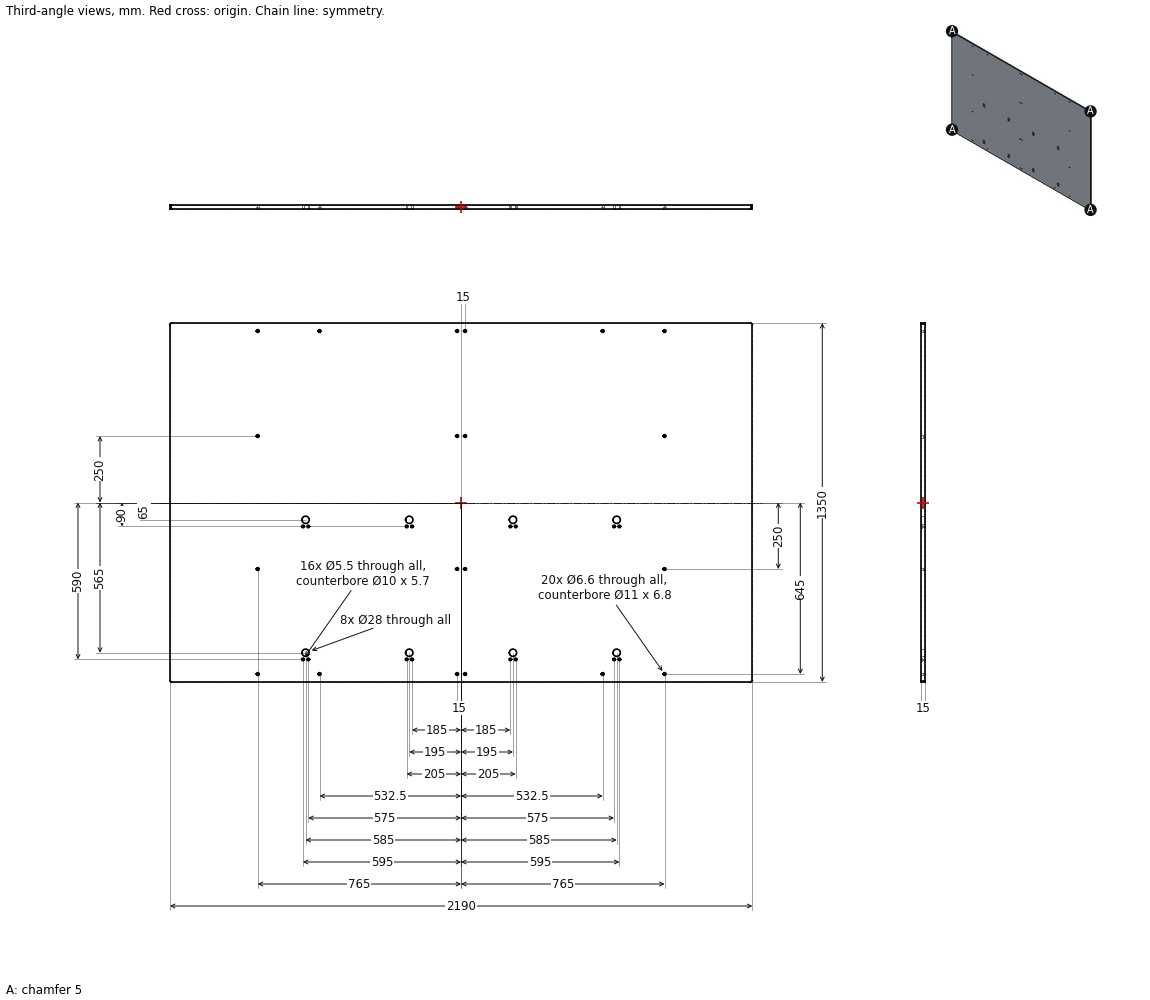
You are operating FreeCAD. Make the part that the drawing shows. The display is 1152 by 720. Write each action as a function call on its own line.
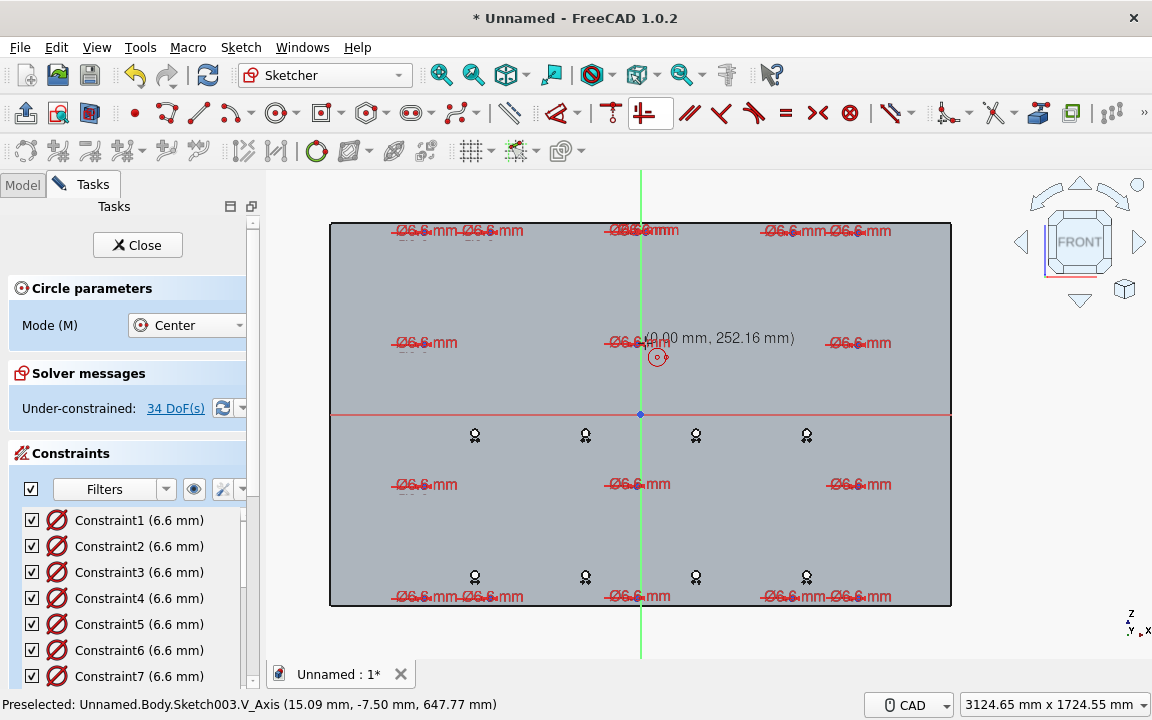
scroll(645, 344, up, 7)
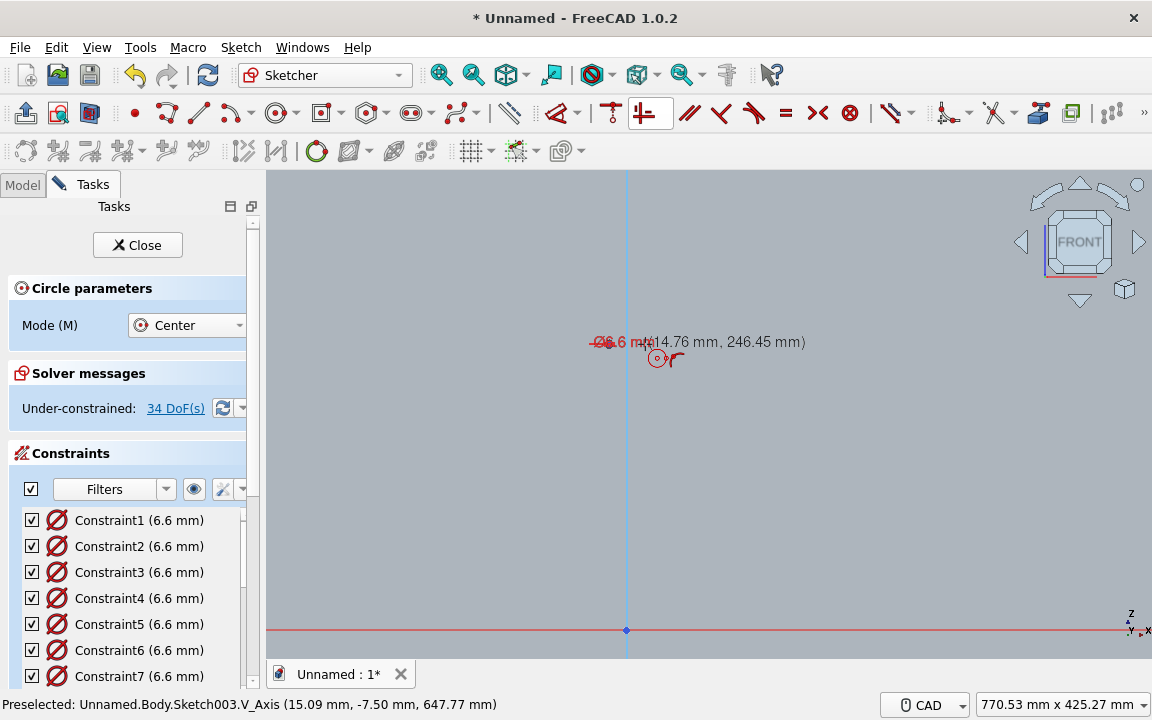
click(644, 343)
move(647, 340)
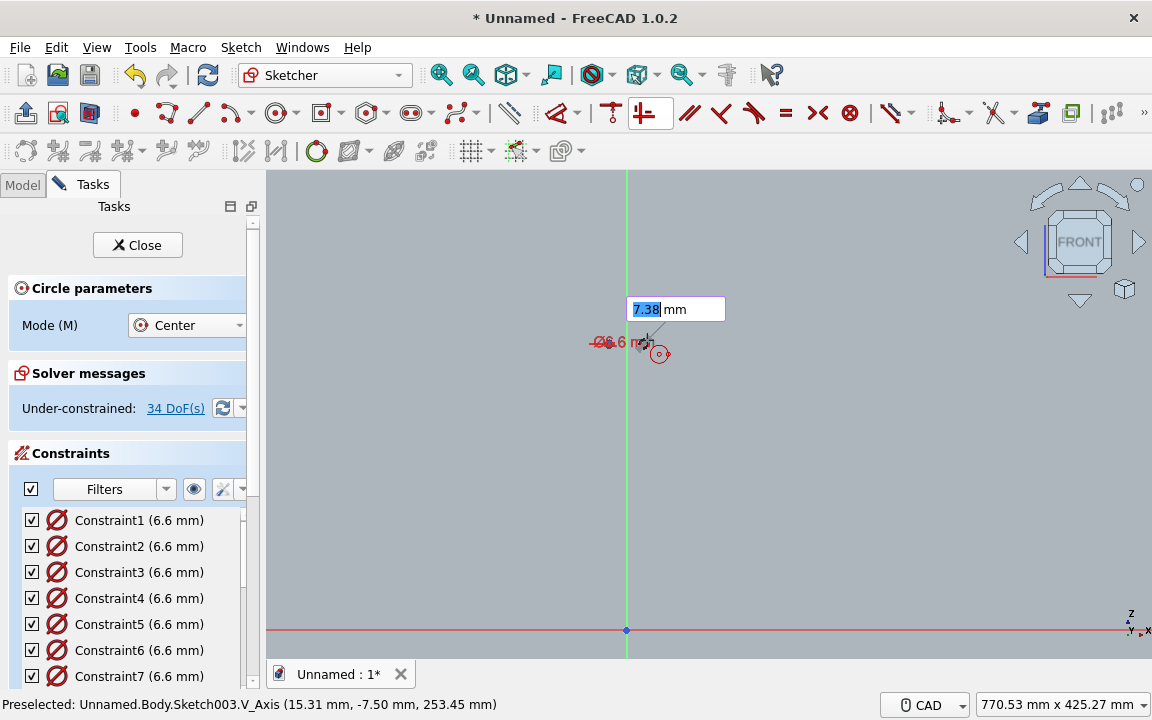
text(6.6)
key(Return)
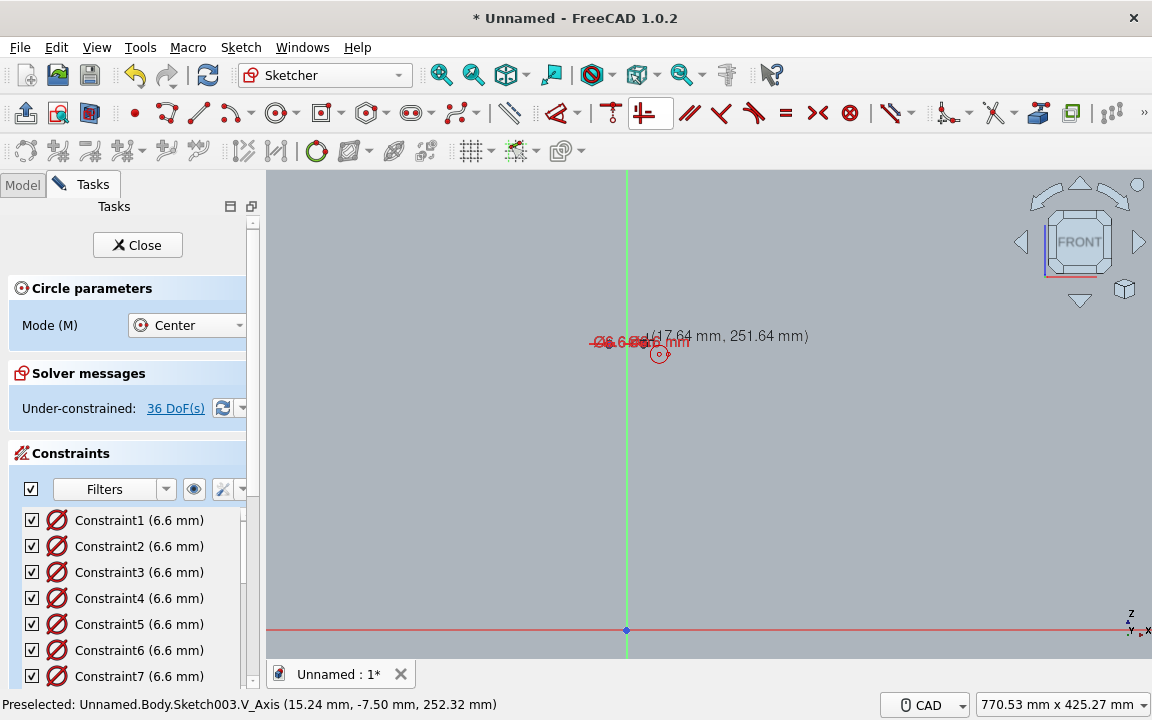
scroll(644, 360, down, 8)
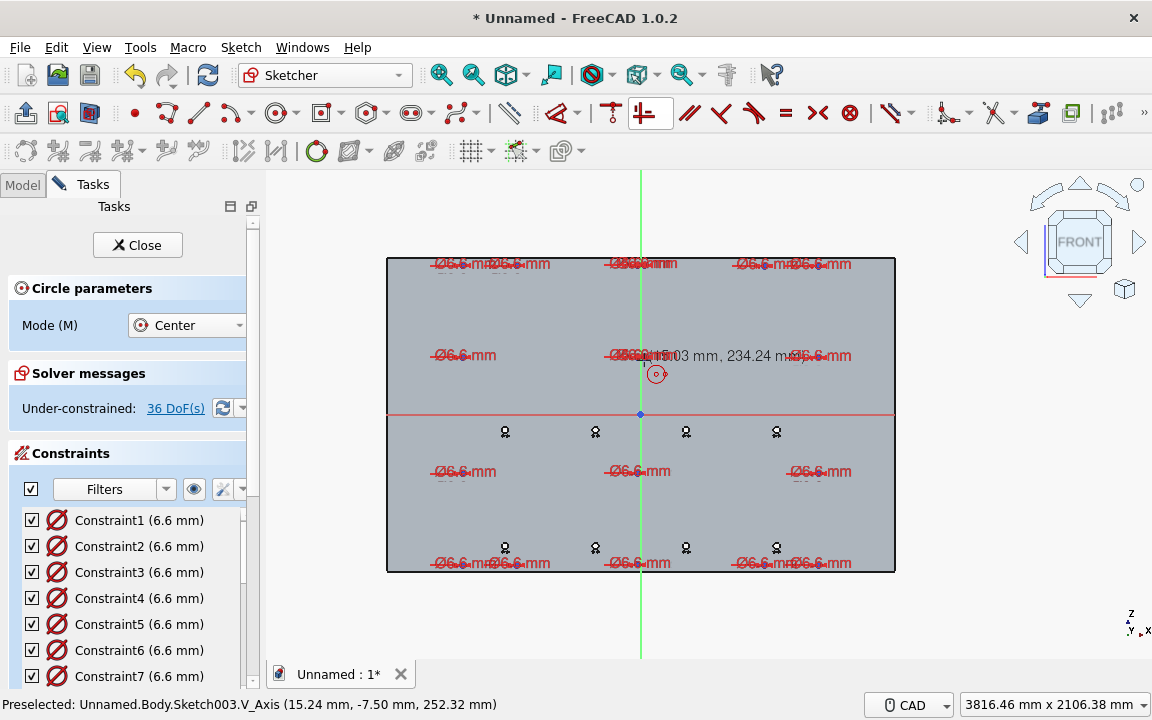
scroll(644, 473, up, 17)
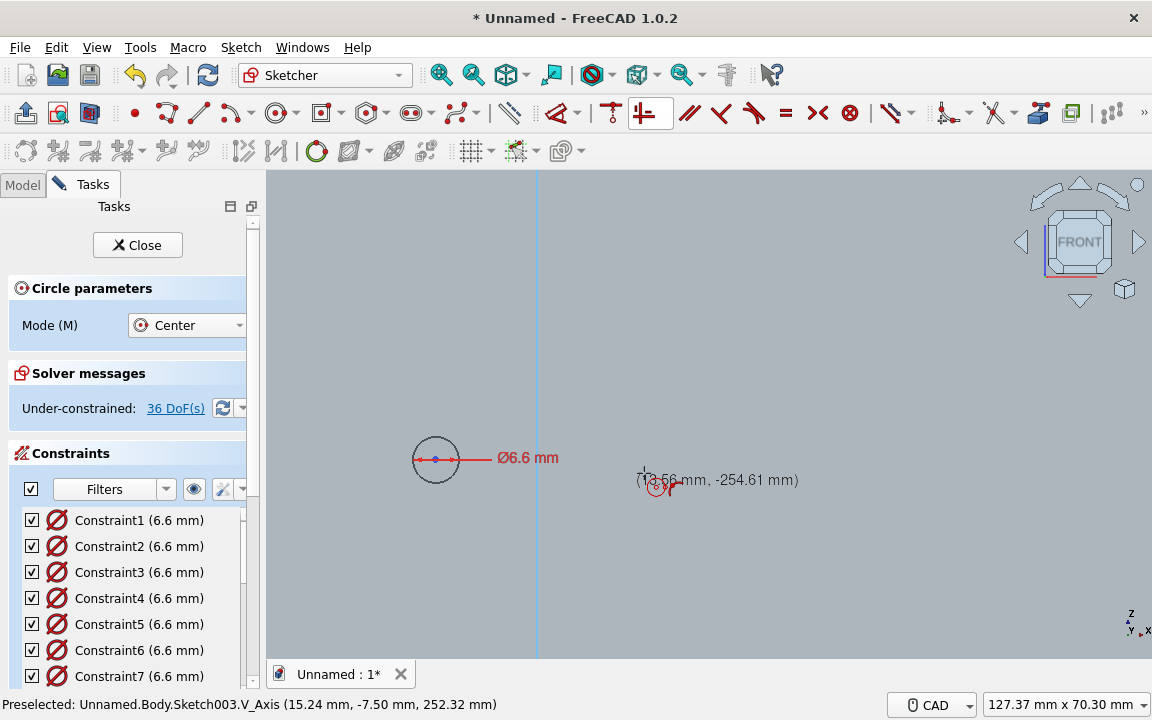
scroll(645, 487, down, 16)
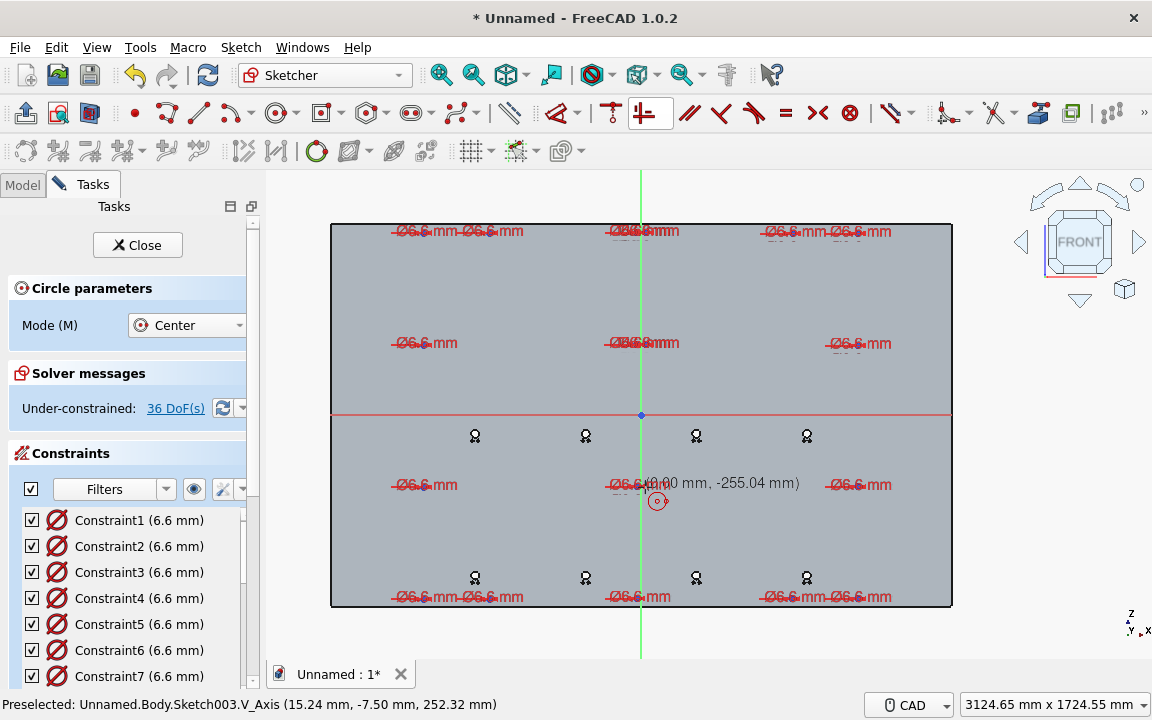
scroll(645, 486, up, 7)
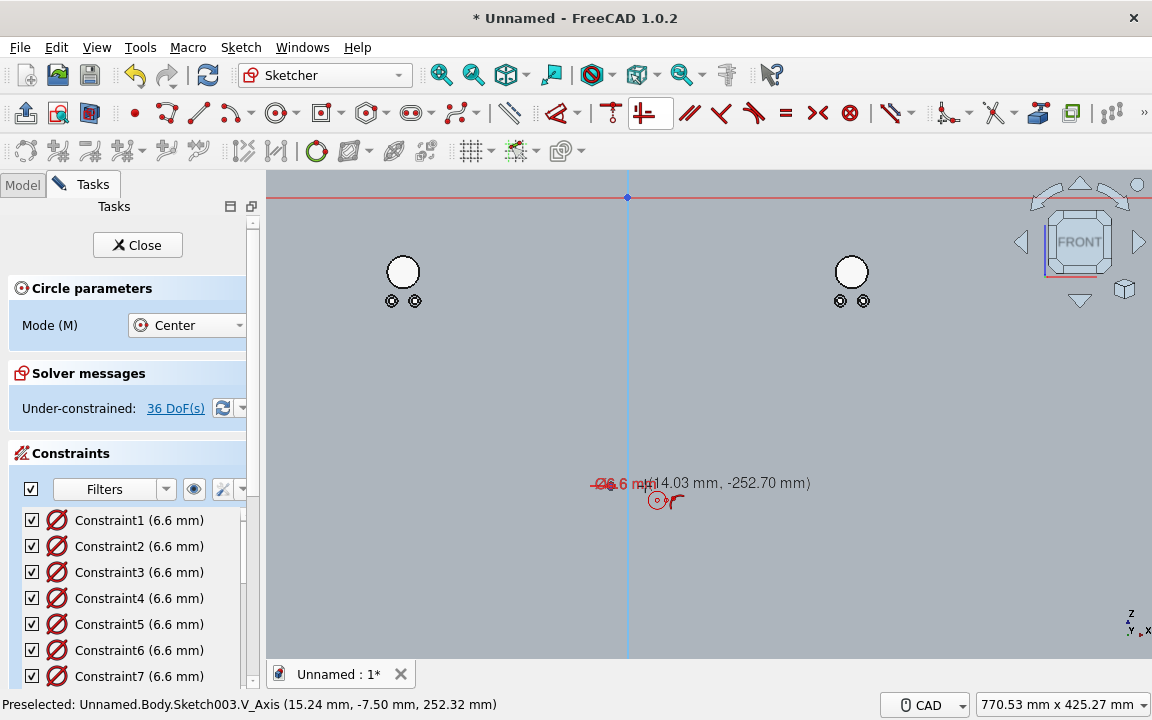
click(645, 485)
move(647, 482)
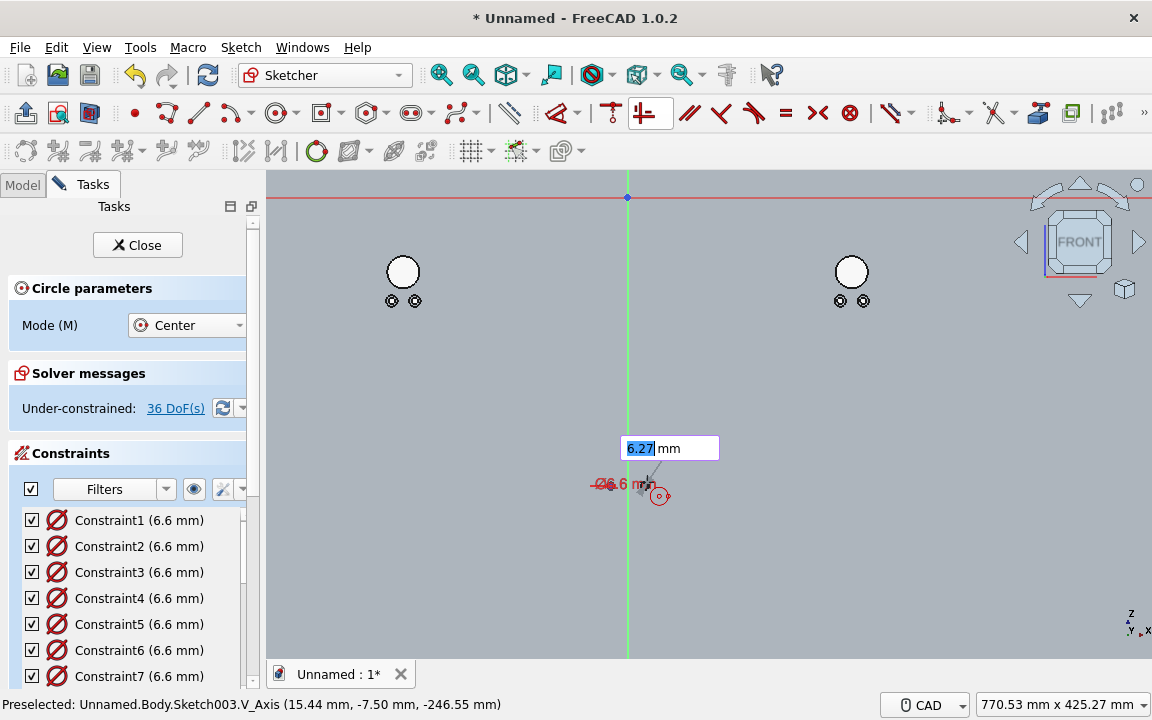
text(6.6)
key(Return)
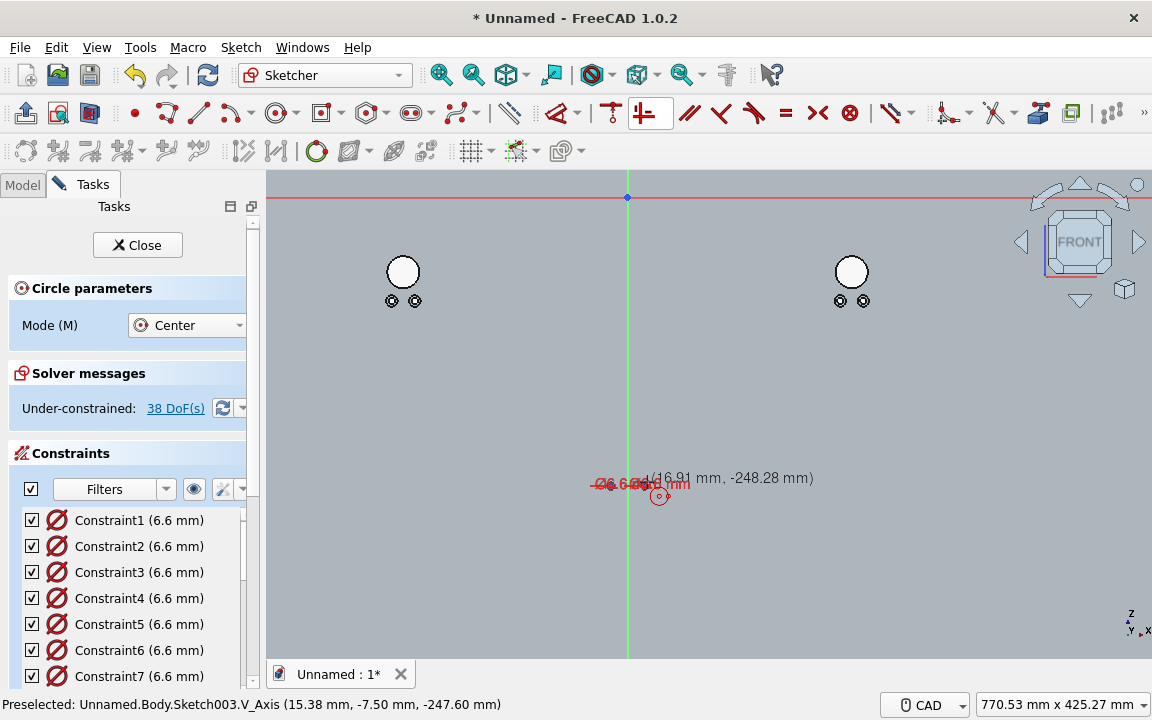
scroll(644, 469, down, 8)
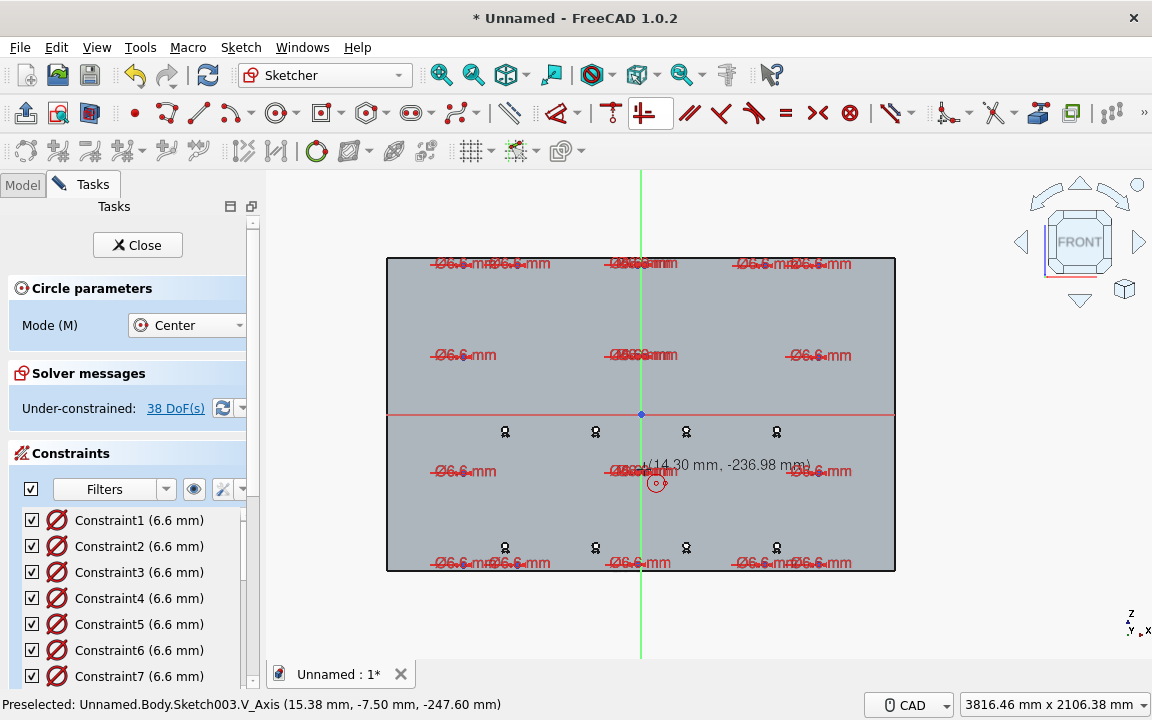
scroll(645, 564, up, 17)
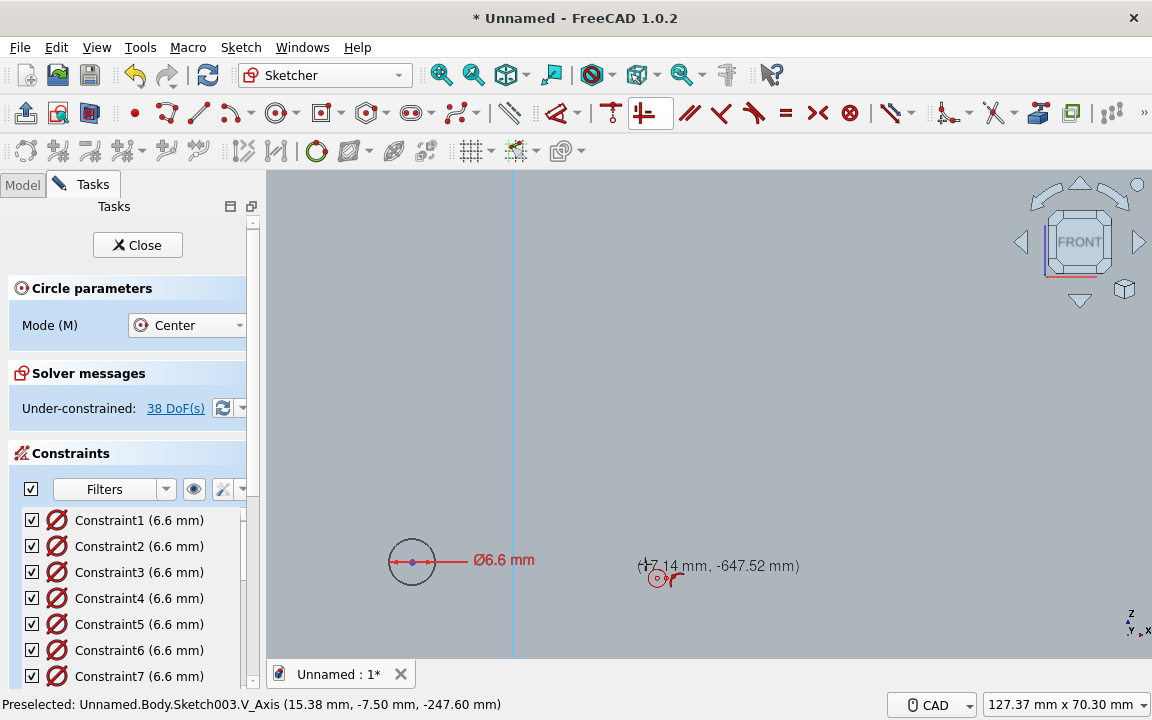
scroll(646, 599, down, 16)